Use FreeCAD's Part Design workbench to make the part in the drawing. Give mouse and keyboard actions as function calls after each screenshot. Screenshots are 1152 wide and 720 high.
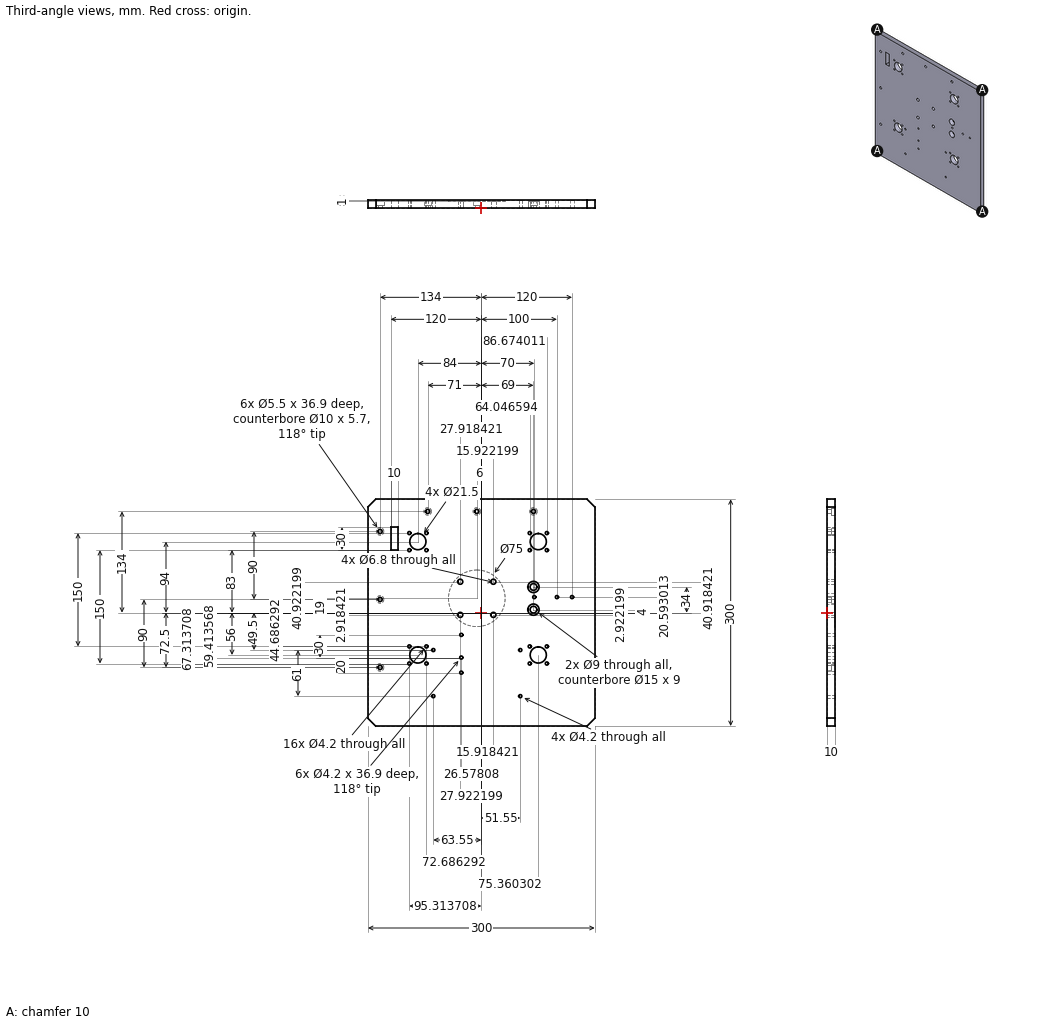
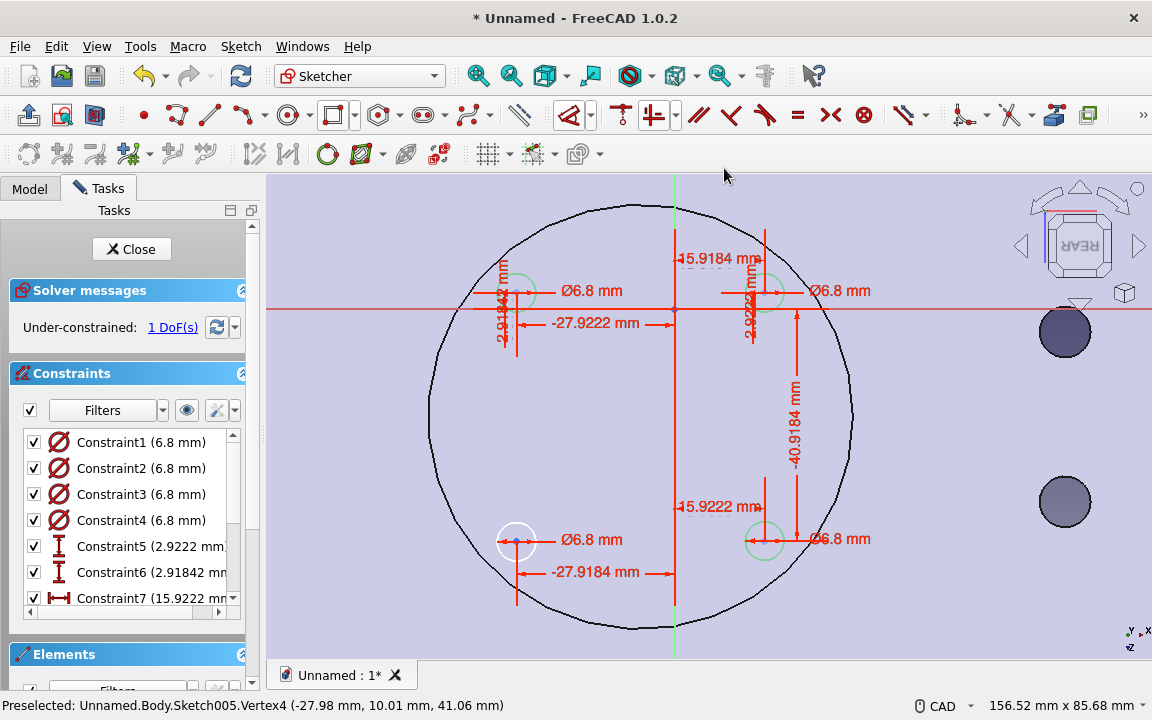
click(517, 542)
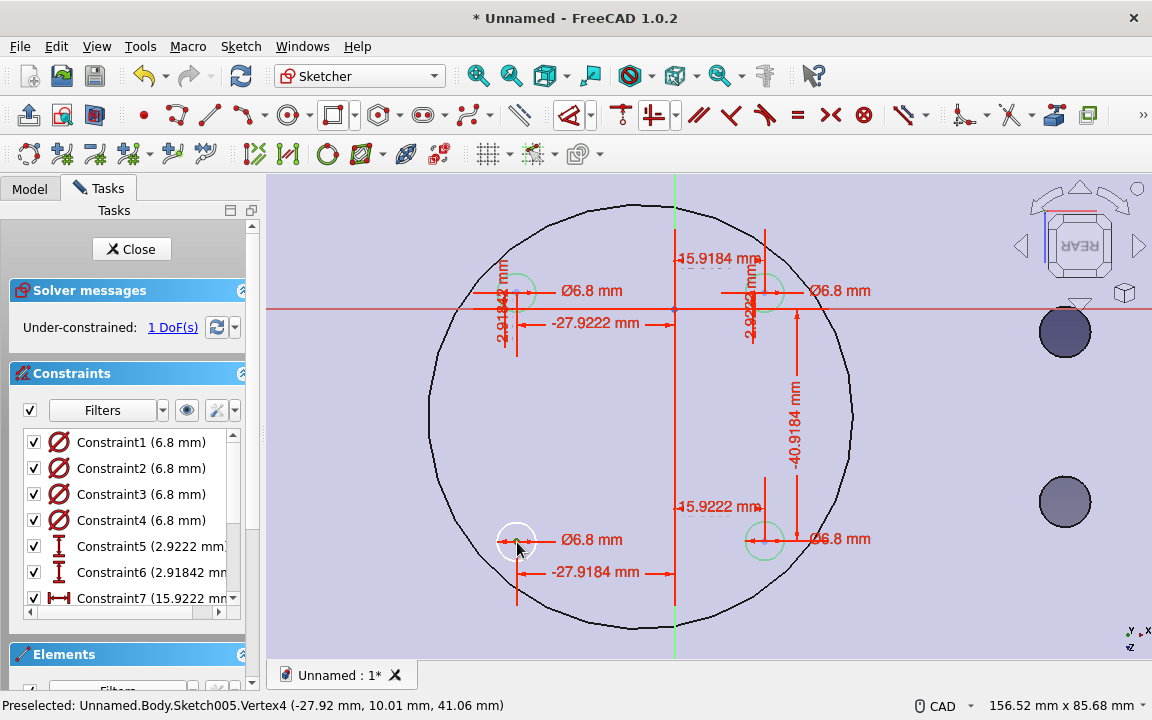
click(590, 116)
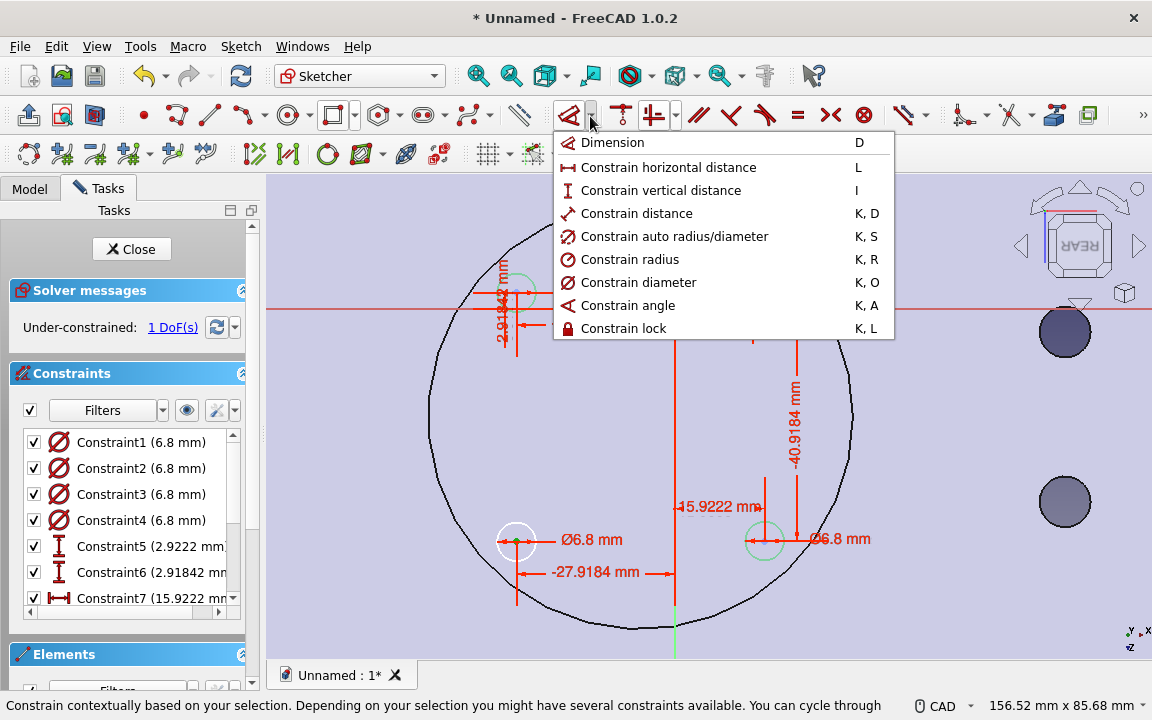
click(724, 190)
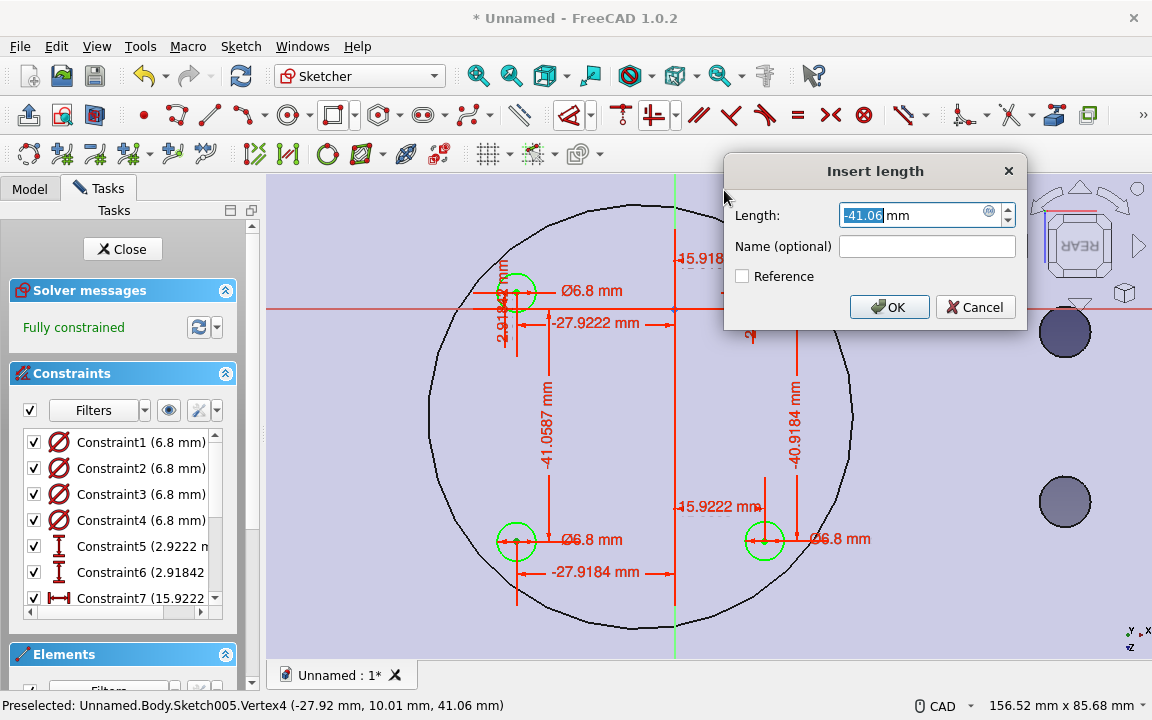
text(-40.922199)
key(Return)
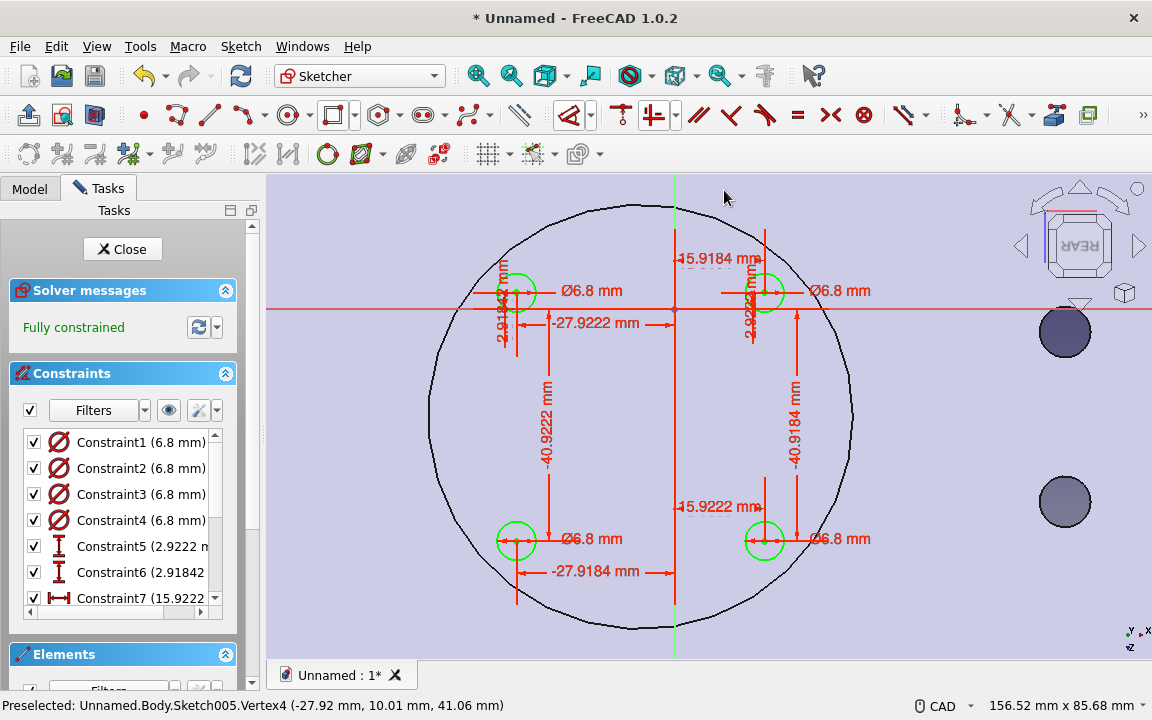
click(123, 249)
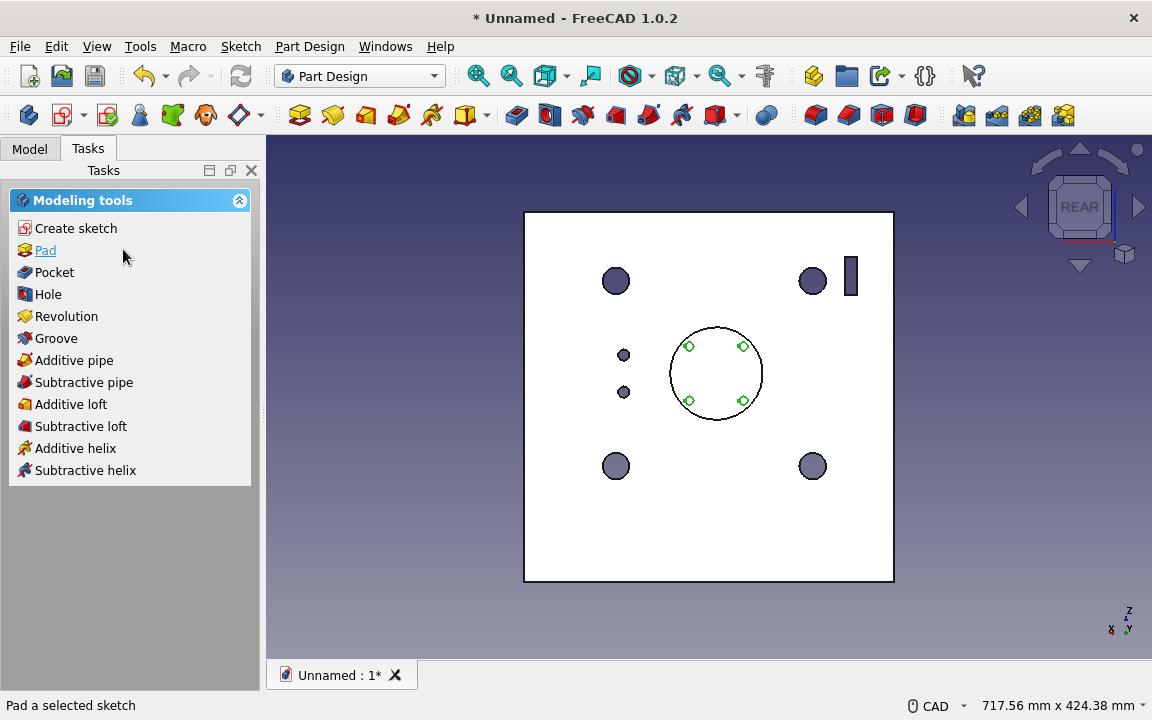
click(550, 116)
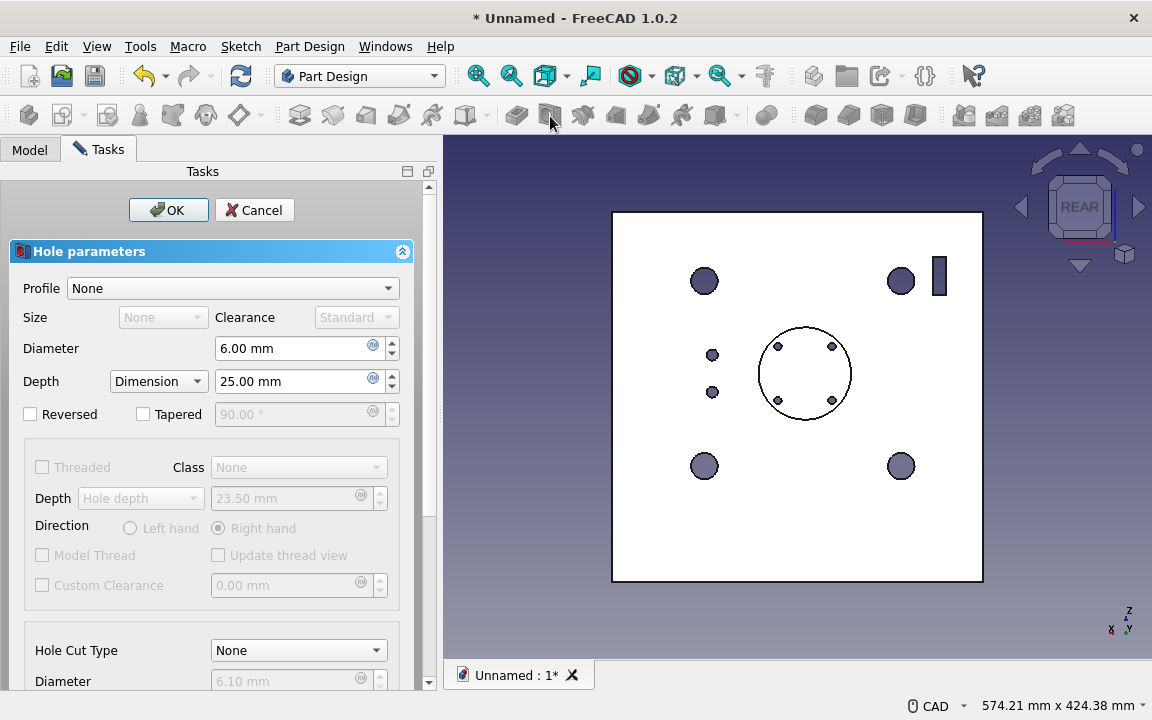
triple_click(300, 348)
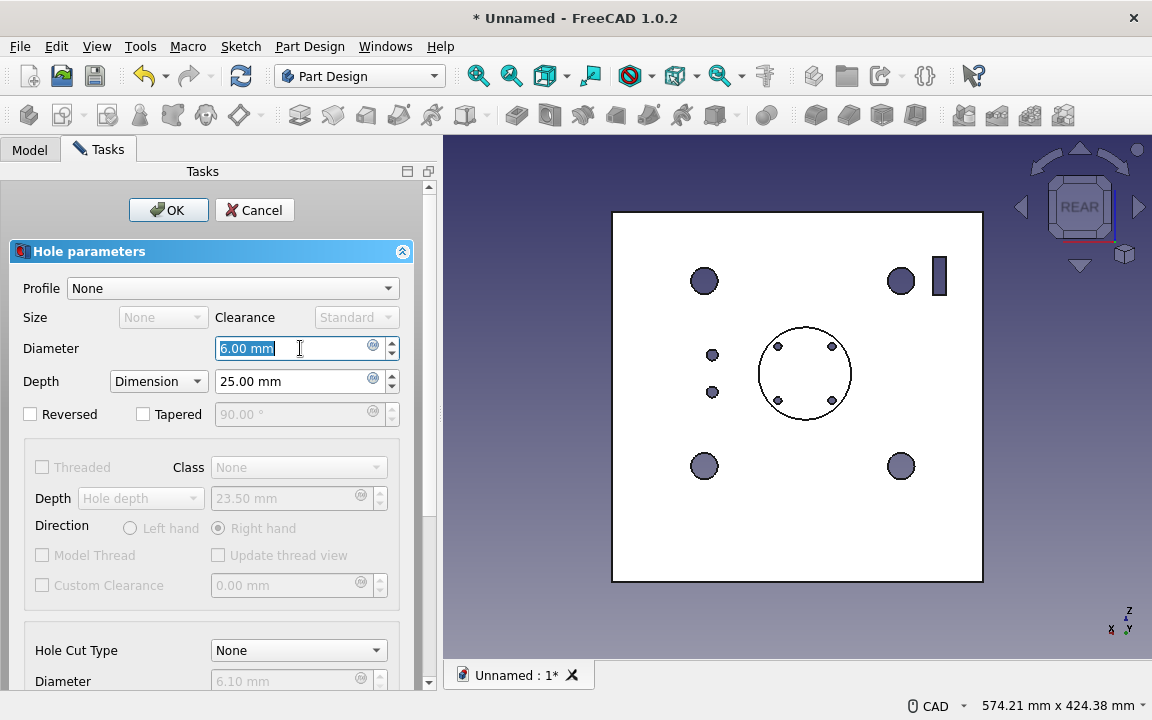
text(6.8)
key(Tab)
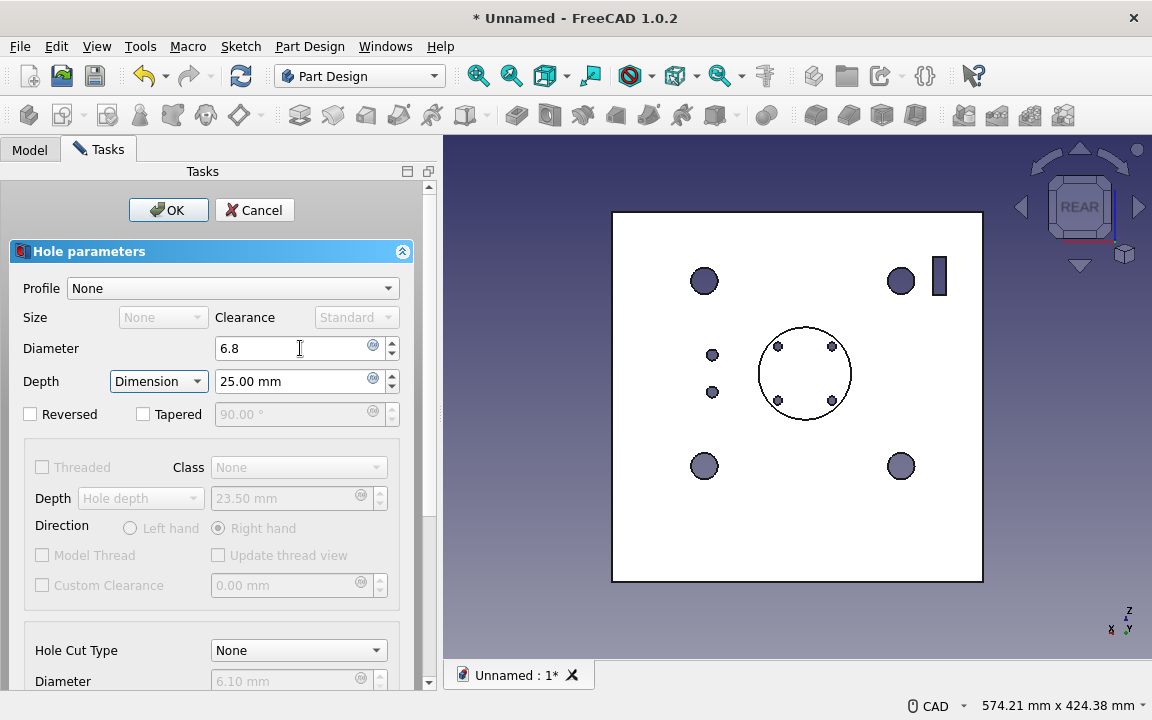
click(160, 382)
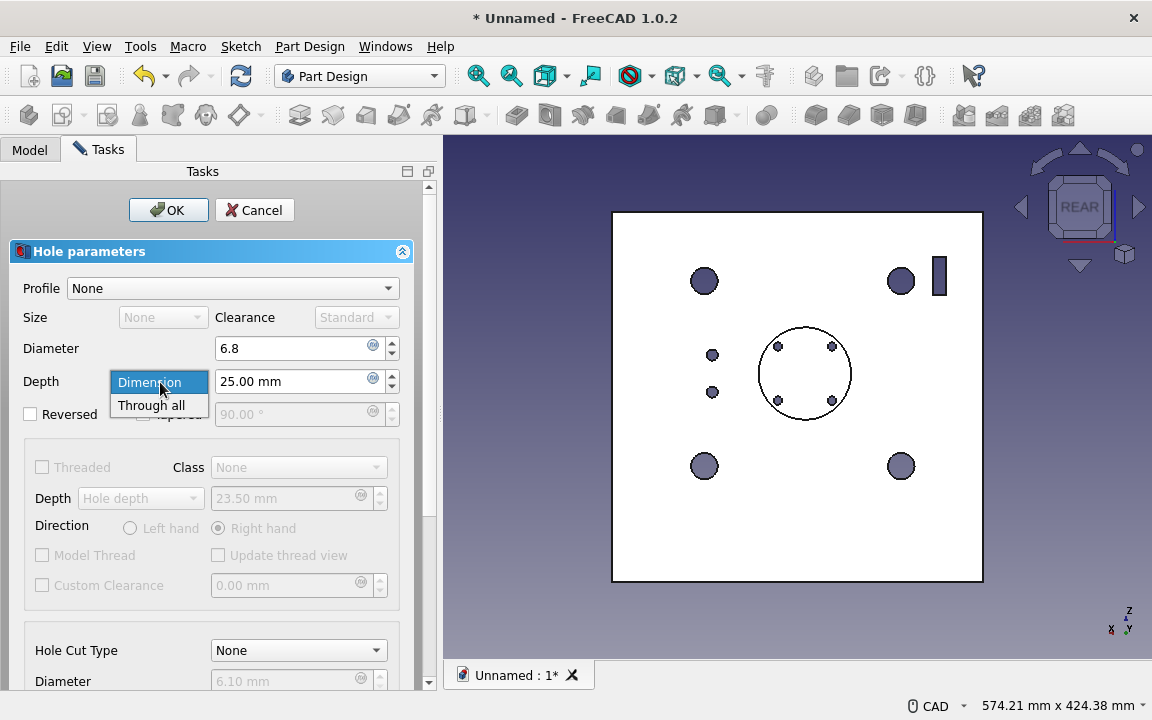
click(158, 406)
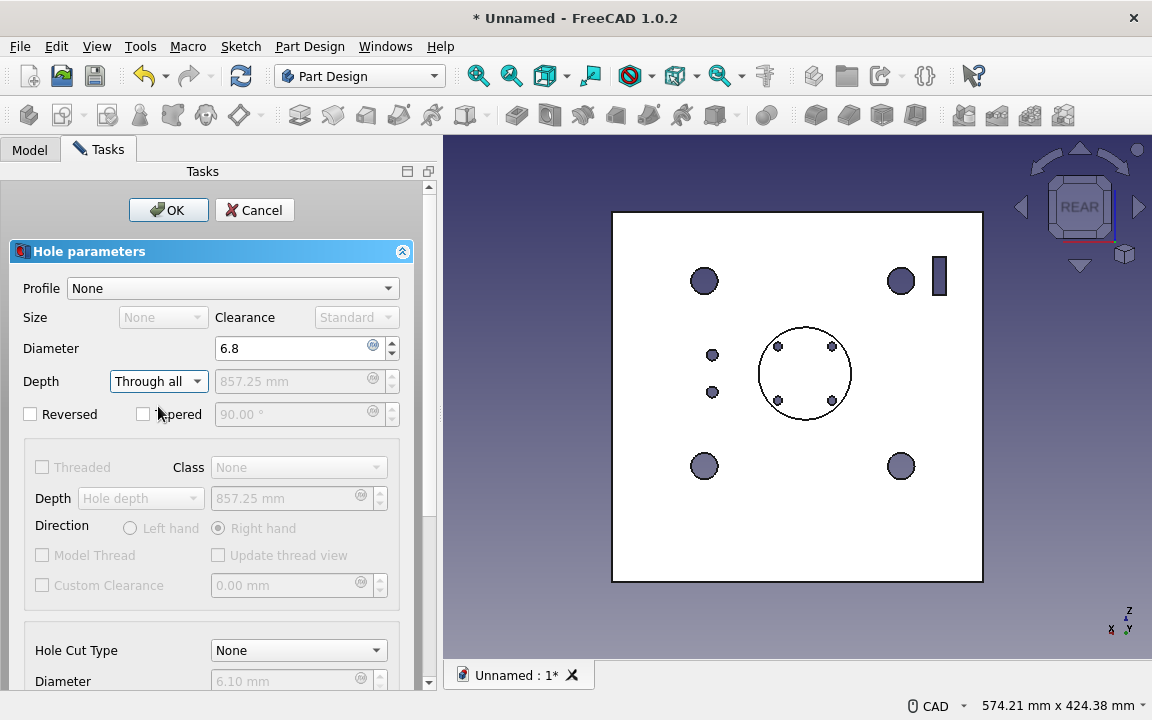
click(169, 210)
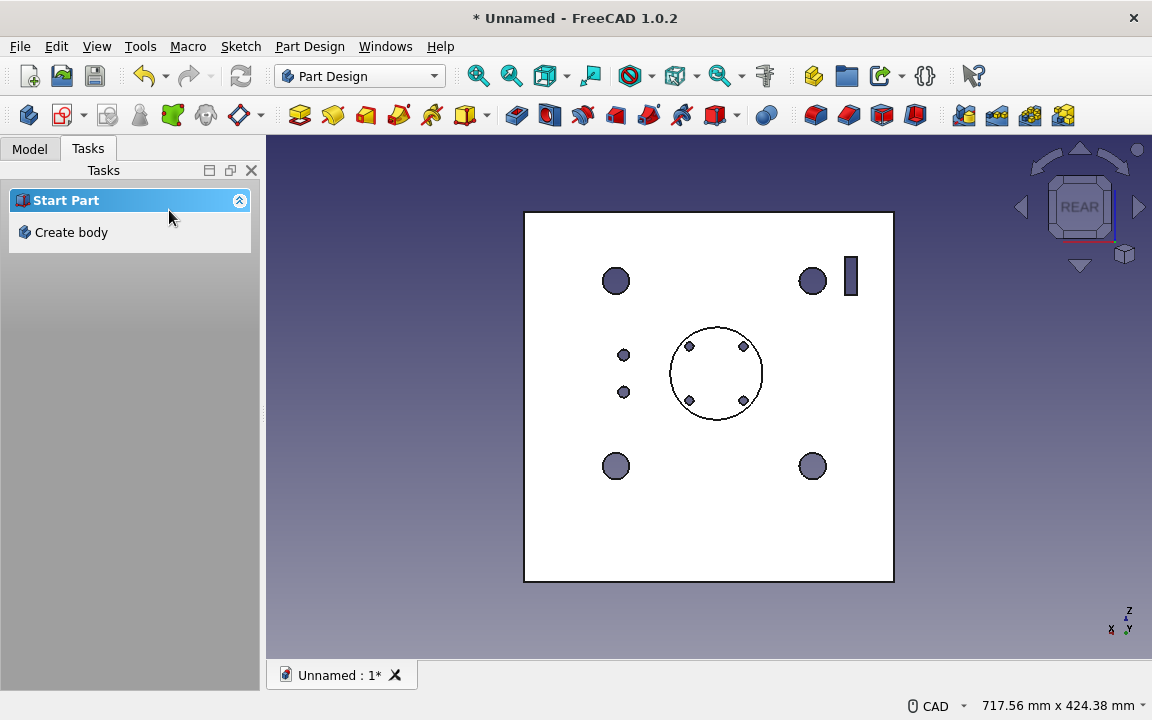
key(0)